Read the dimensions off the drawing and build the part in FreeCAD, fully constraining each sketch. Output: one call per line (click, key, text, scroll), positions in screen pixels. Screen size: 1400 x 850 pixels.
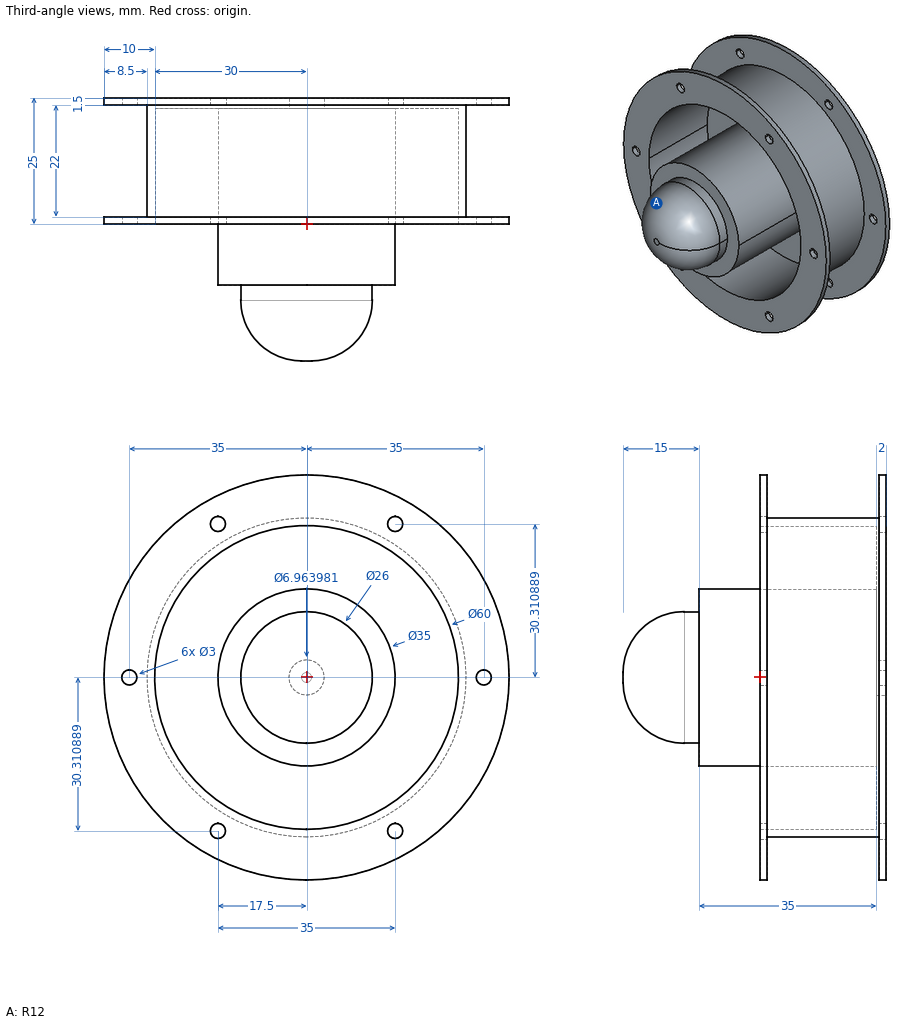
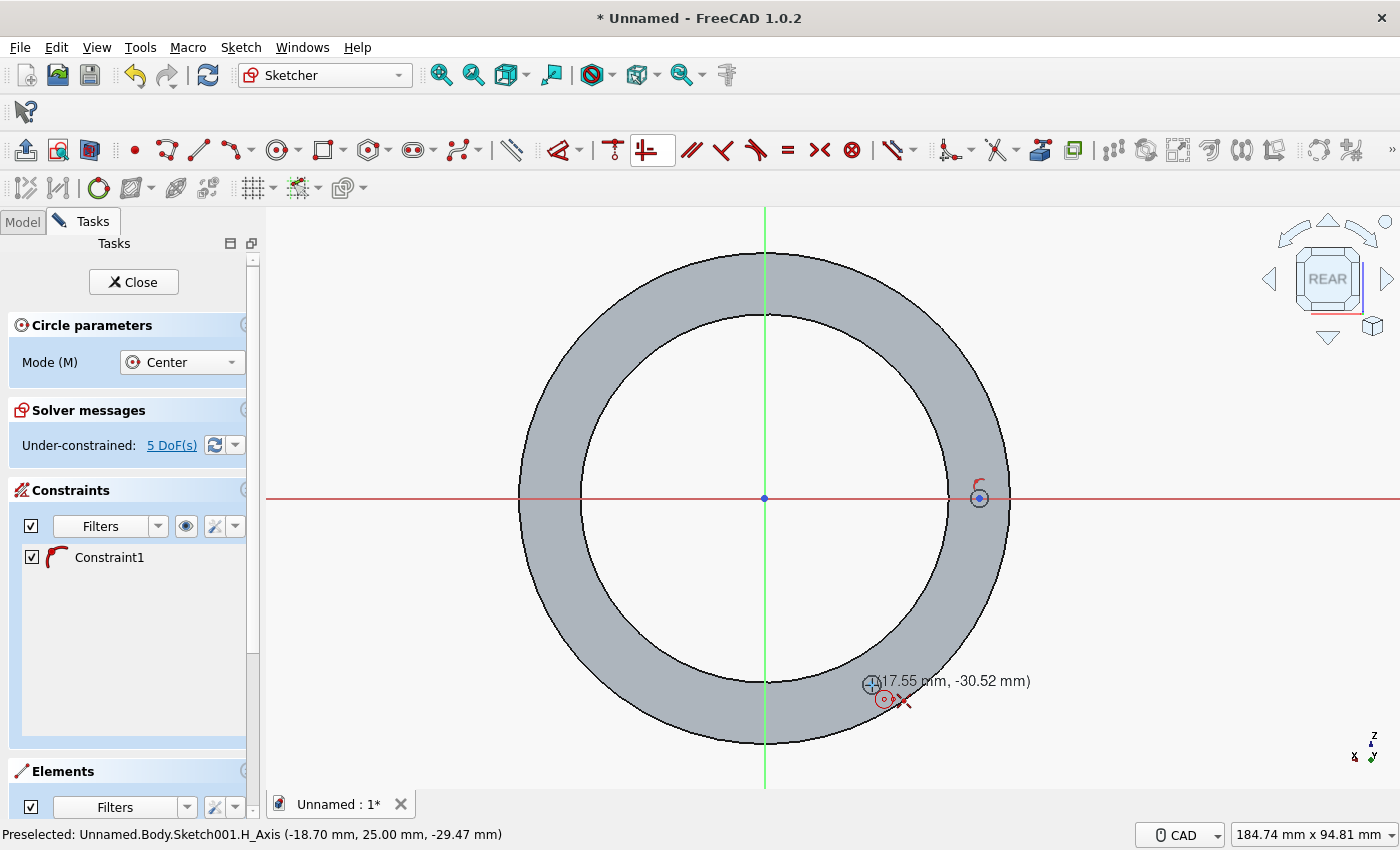
scroll(657, 685, up, 5)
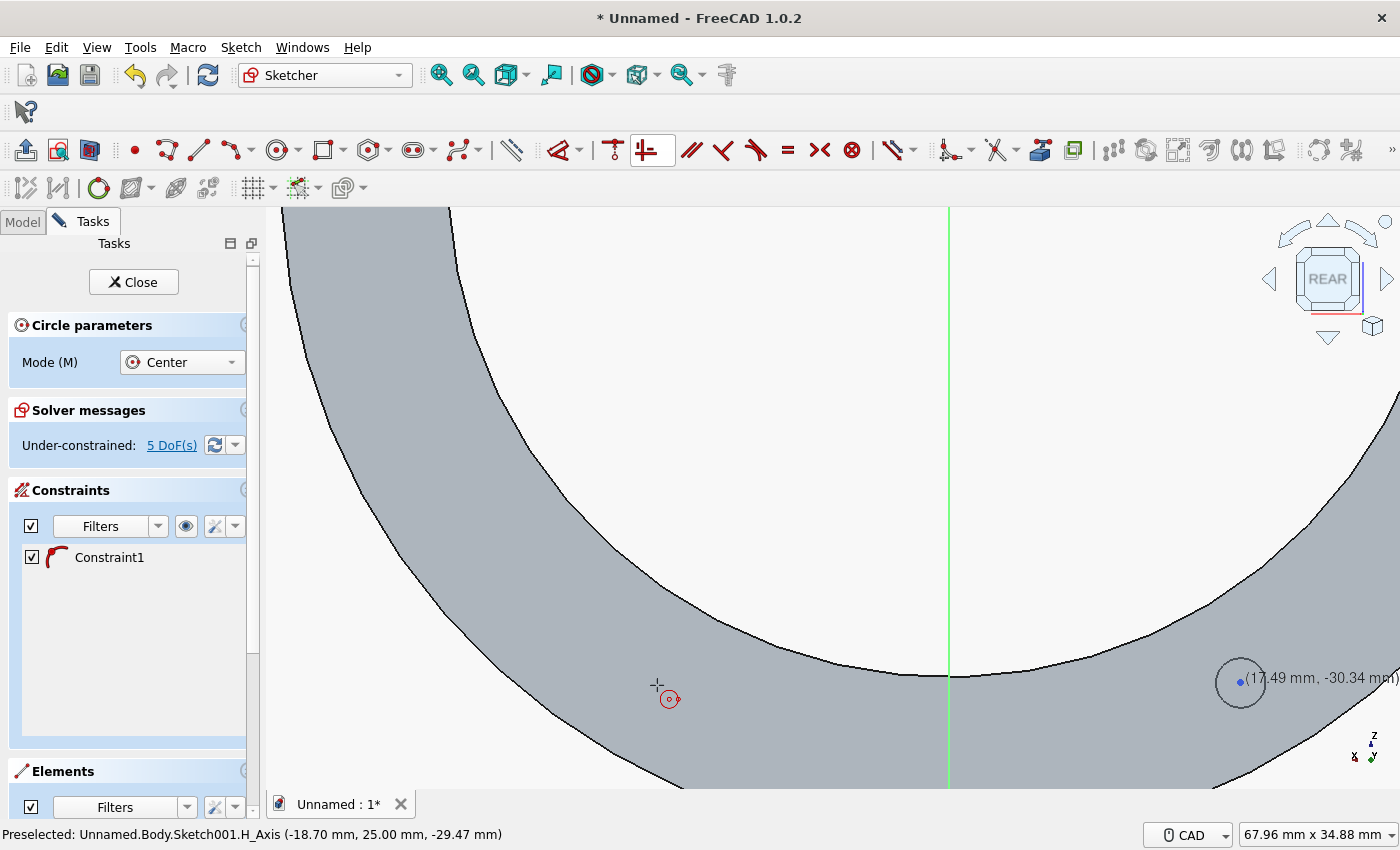
click(657, 682)
click(675, 665)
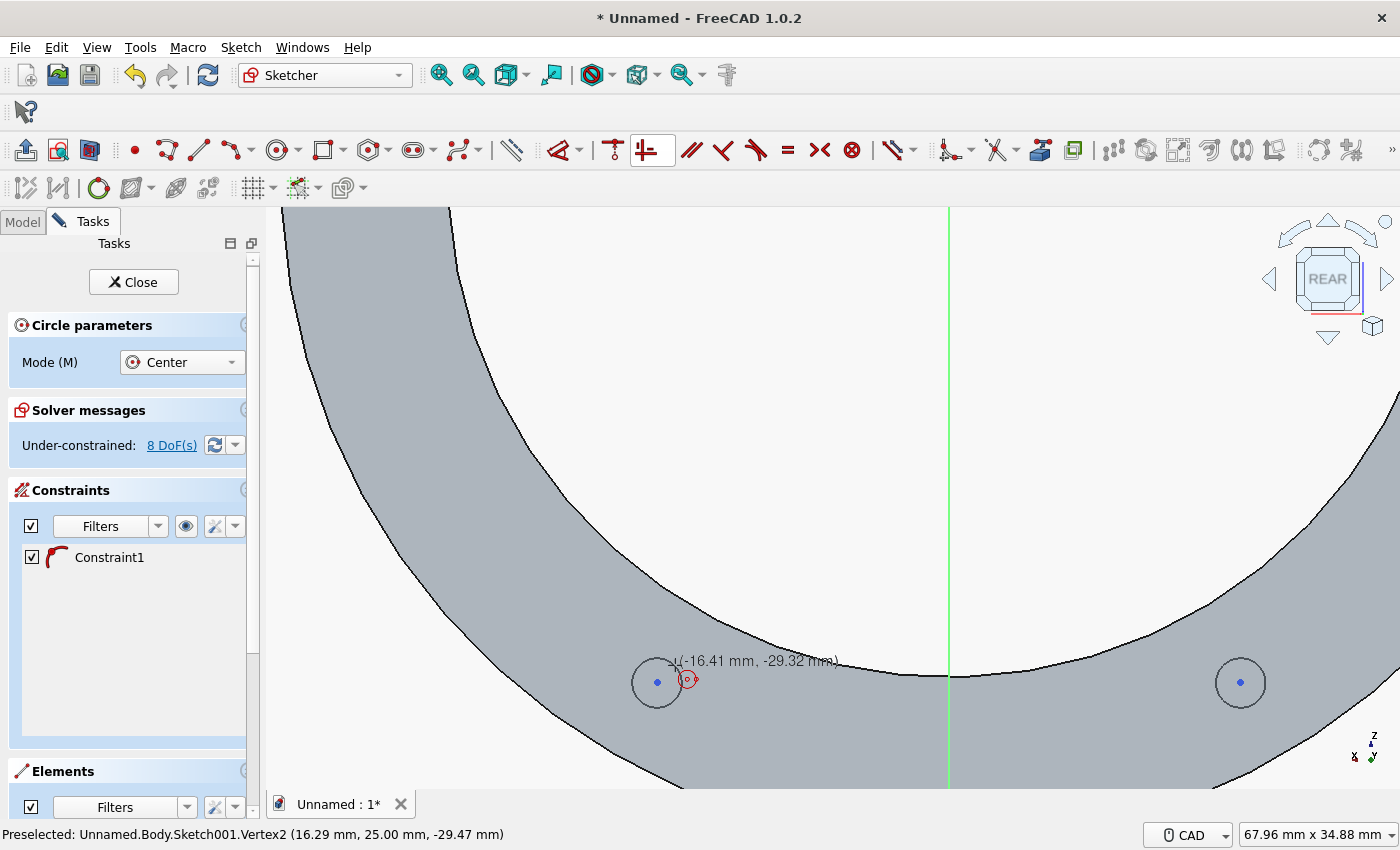
scroll(657, 685, down, 5)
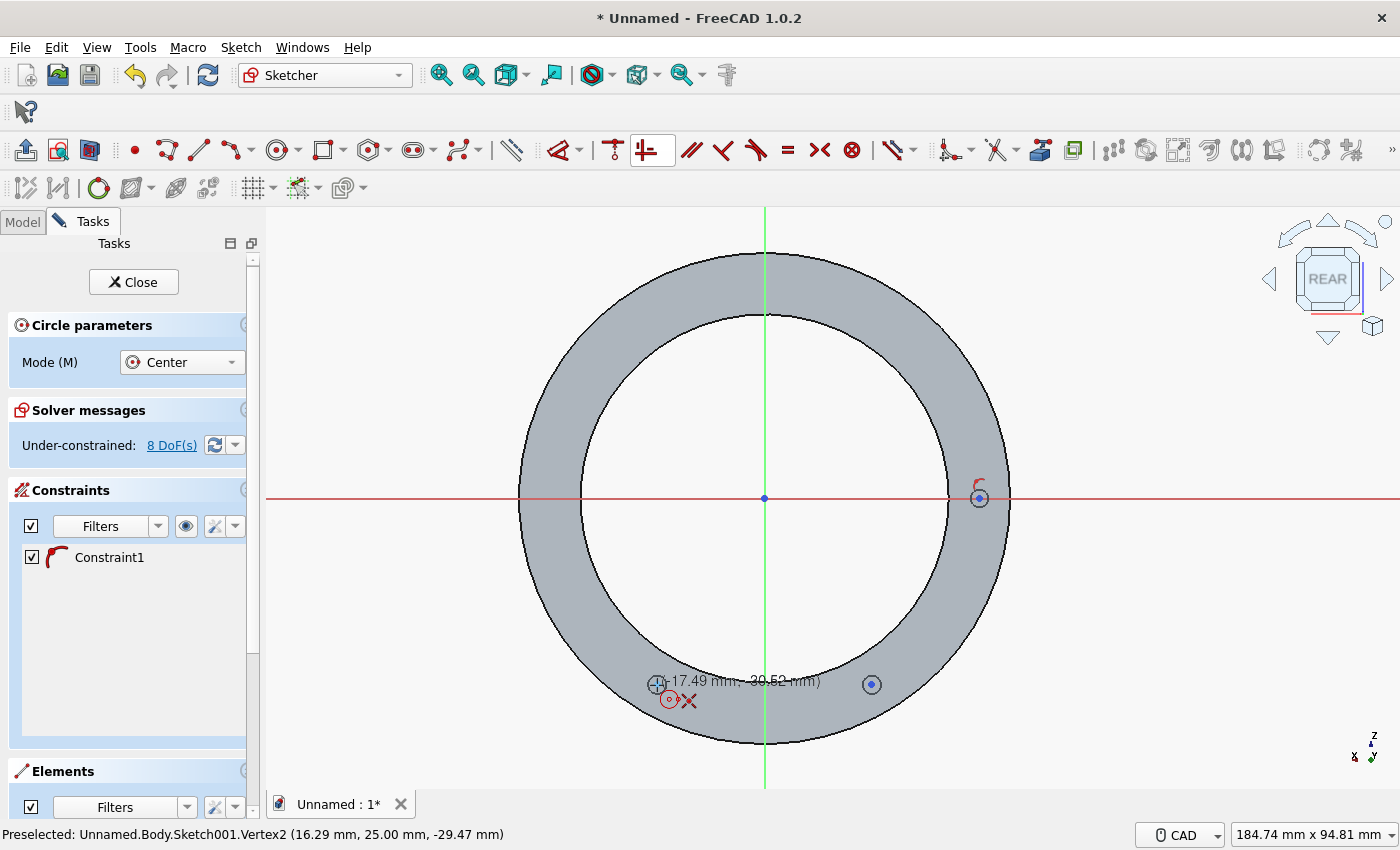
scroll(550, 499, up, 5)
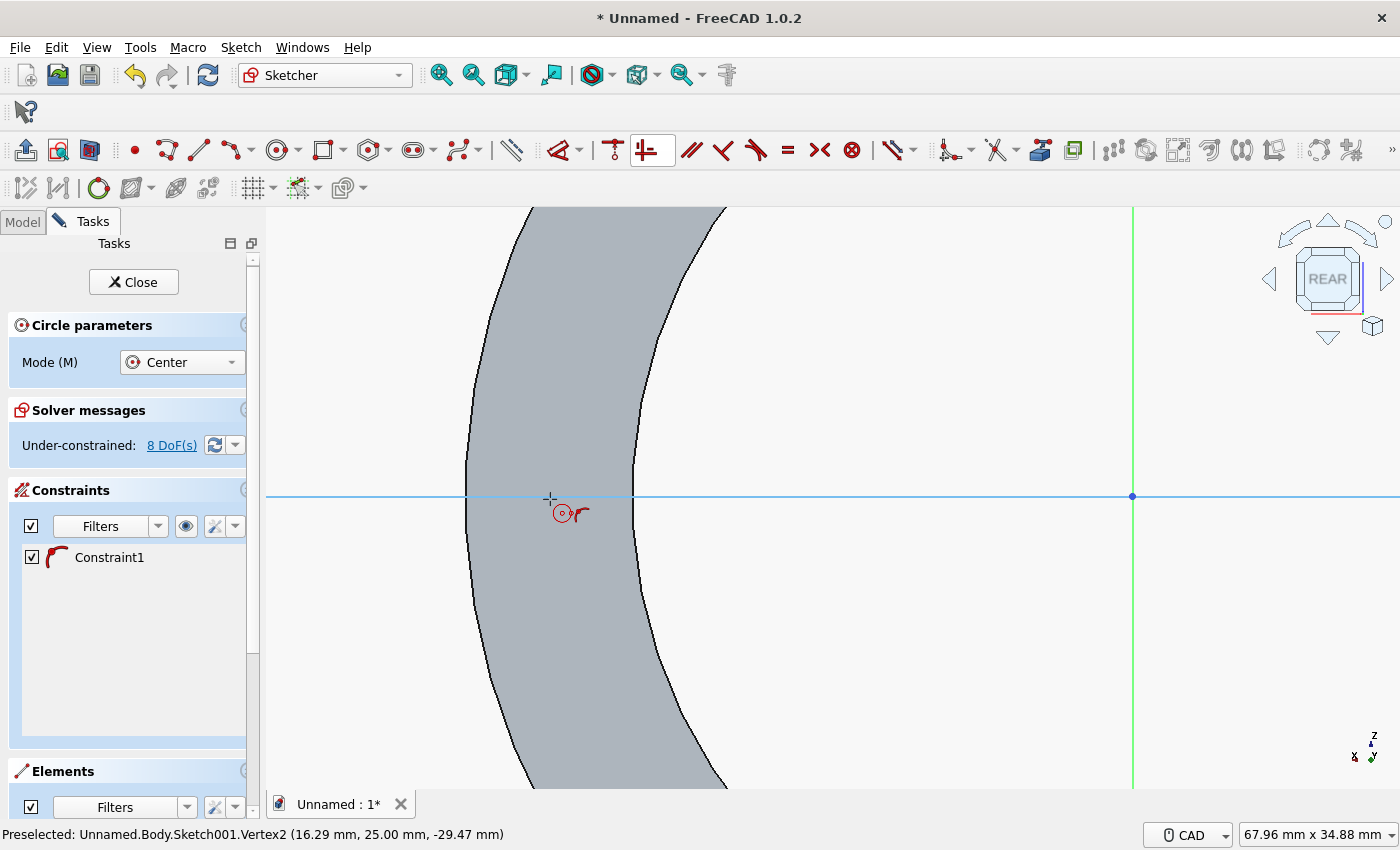
click(549, 497)
click(567, 479)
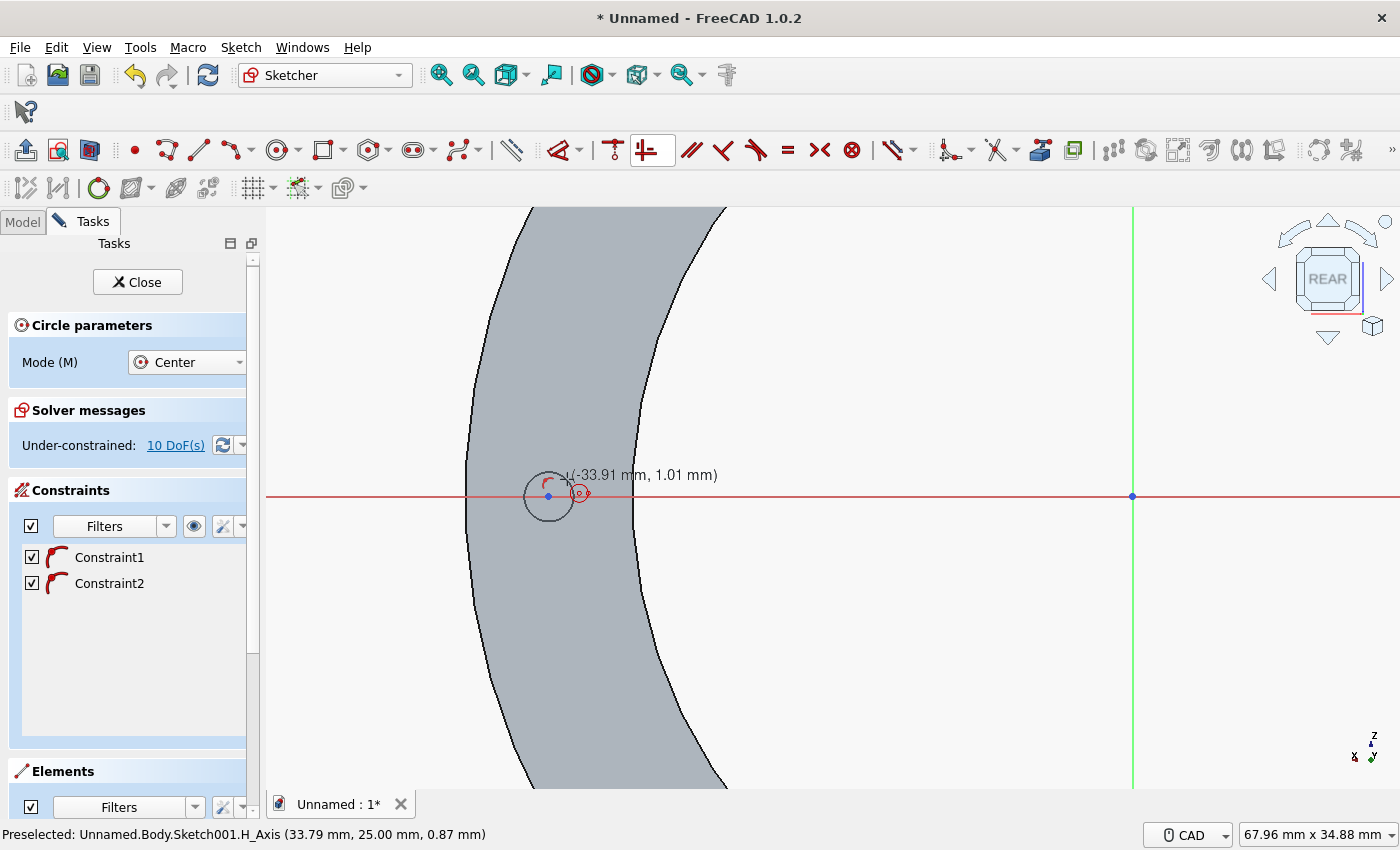
scroll(550, 499, down, 5)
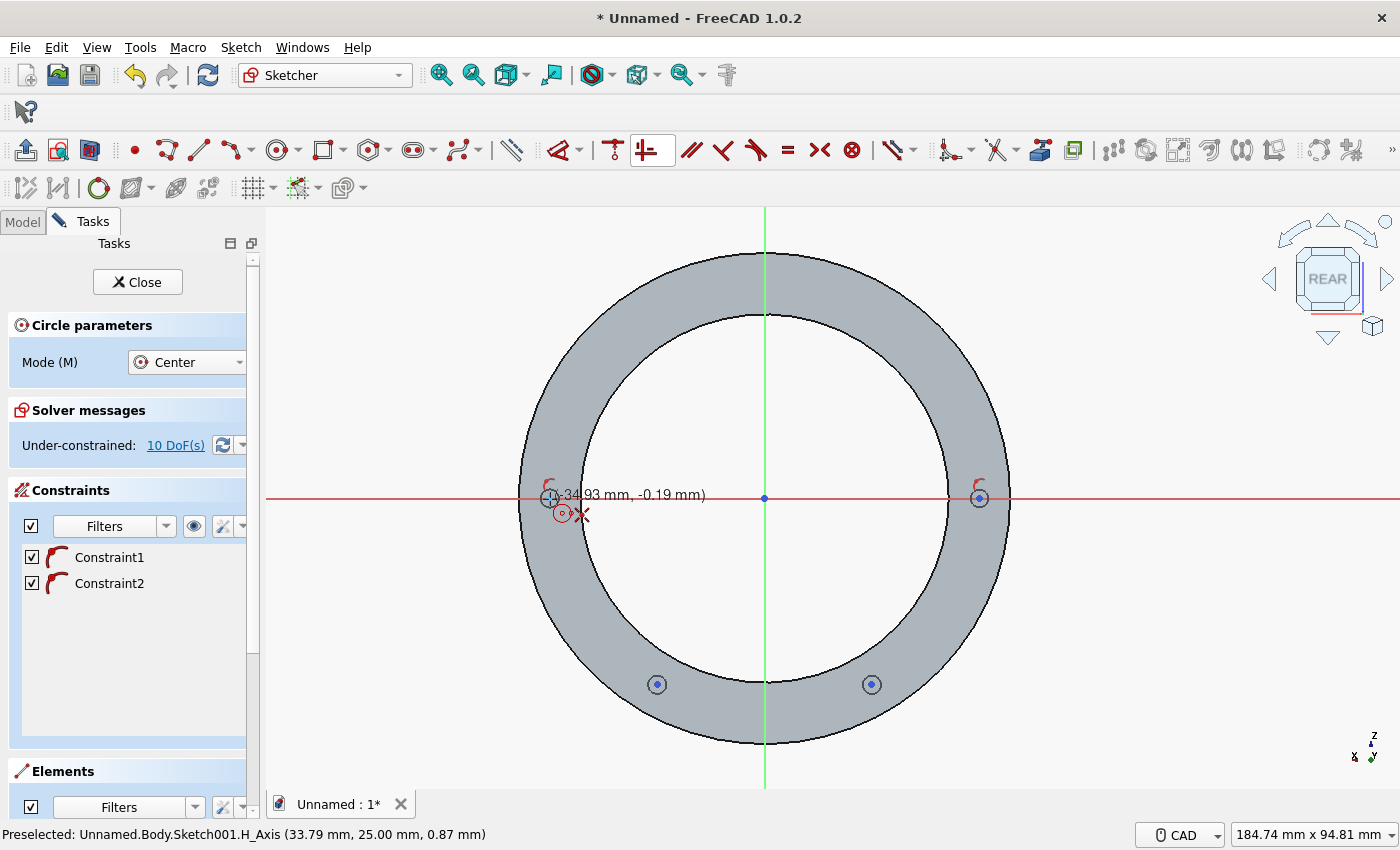
scroll(657, 312, up, 5)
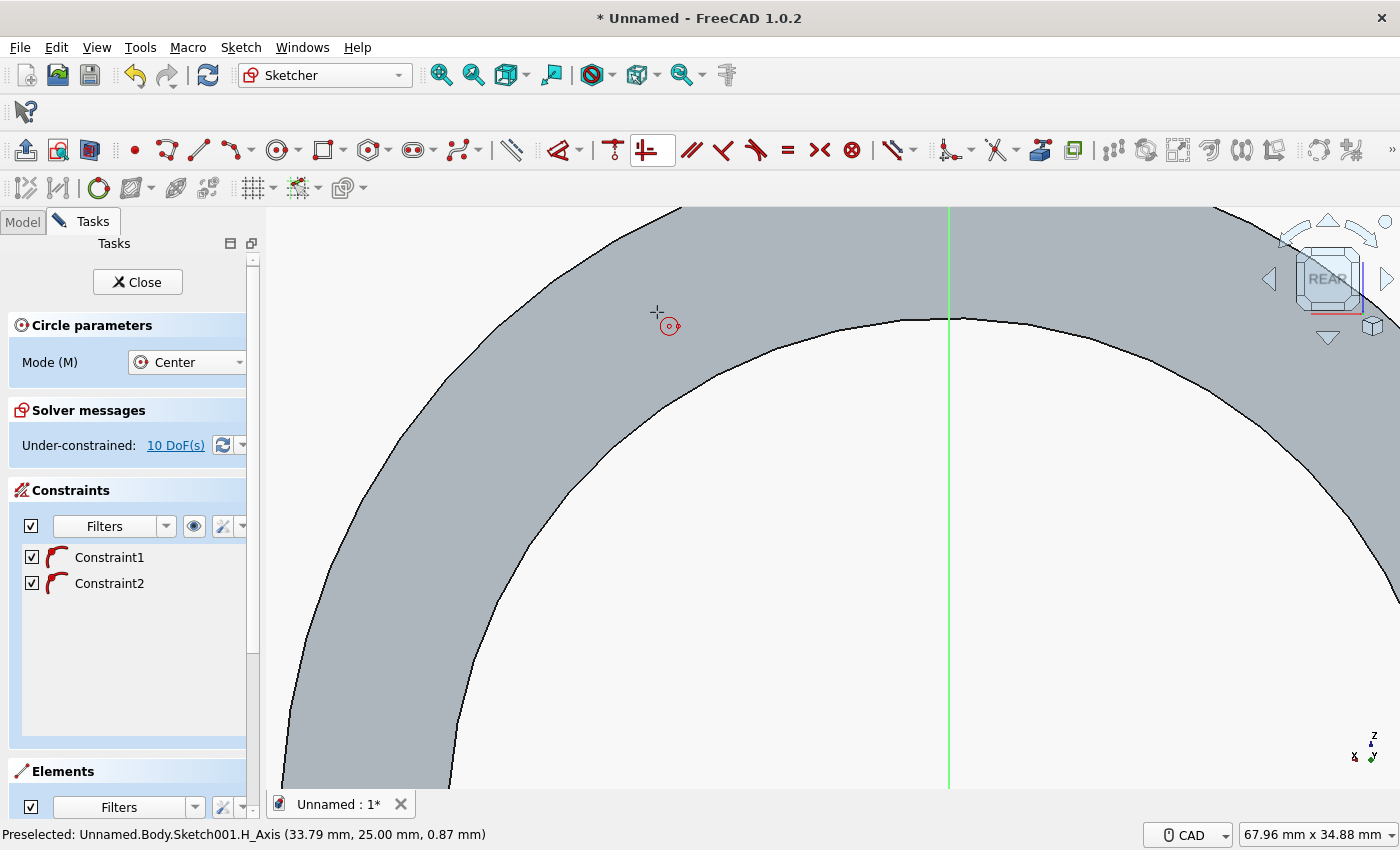
click(657, 313)
click(675, 295)